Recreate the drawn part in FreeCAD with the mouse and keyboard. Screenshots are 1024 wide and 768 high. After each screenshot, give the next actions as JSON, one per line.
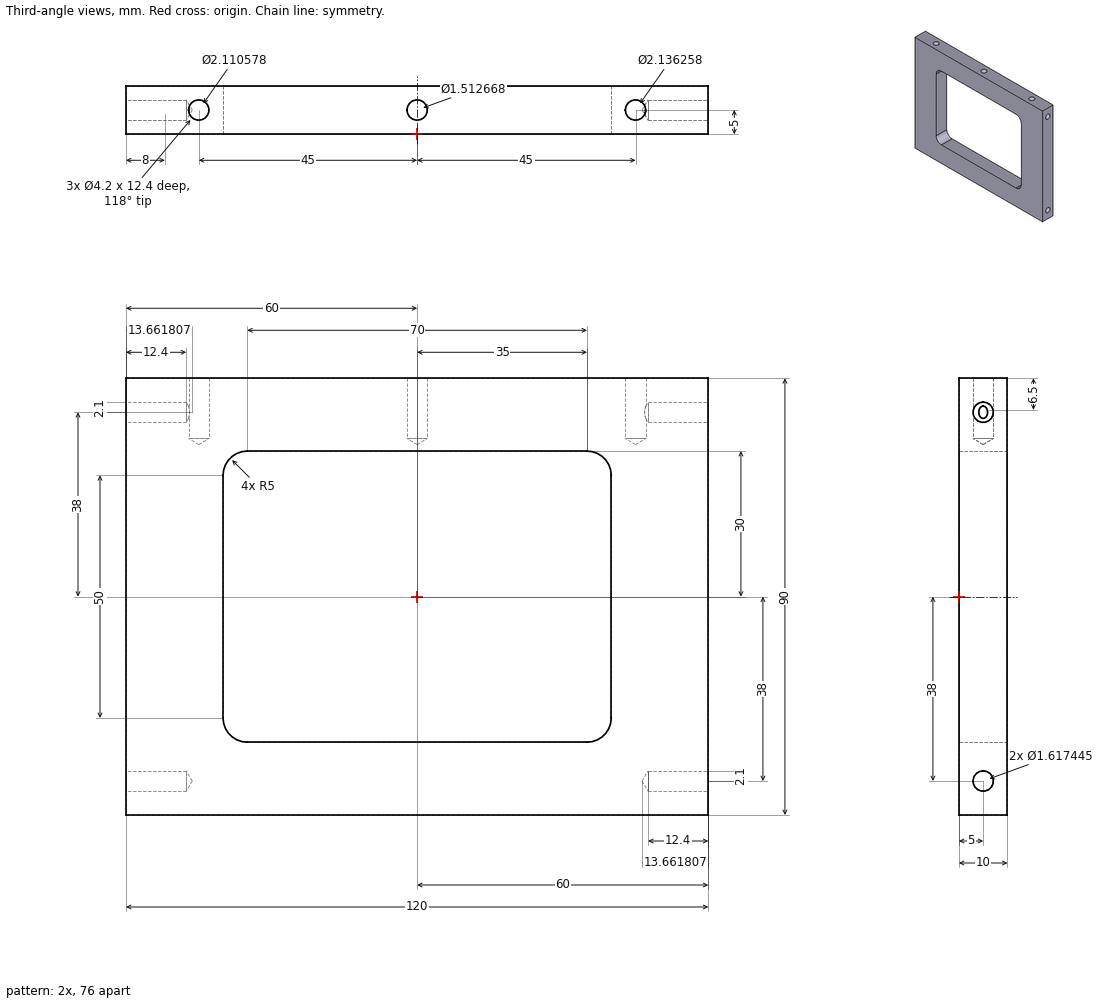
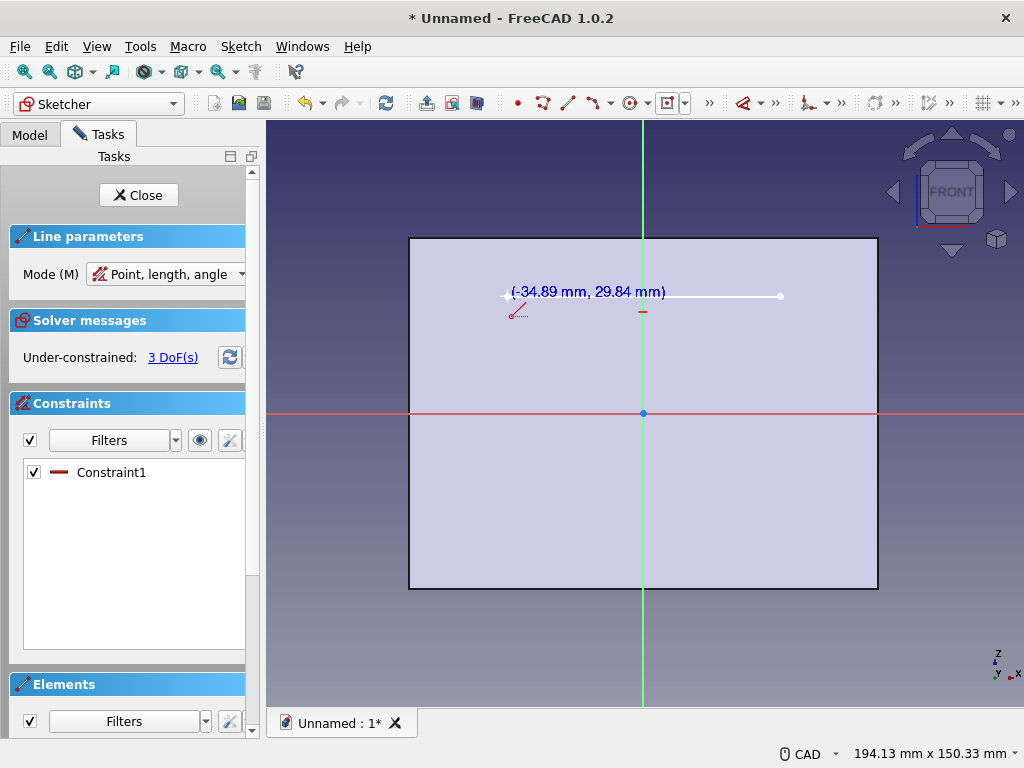
{"action": "left_click", "coordinate": [487, 316]}
{"action": "left_click", "coordinate": [487, 511]}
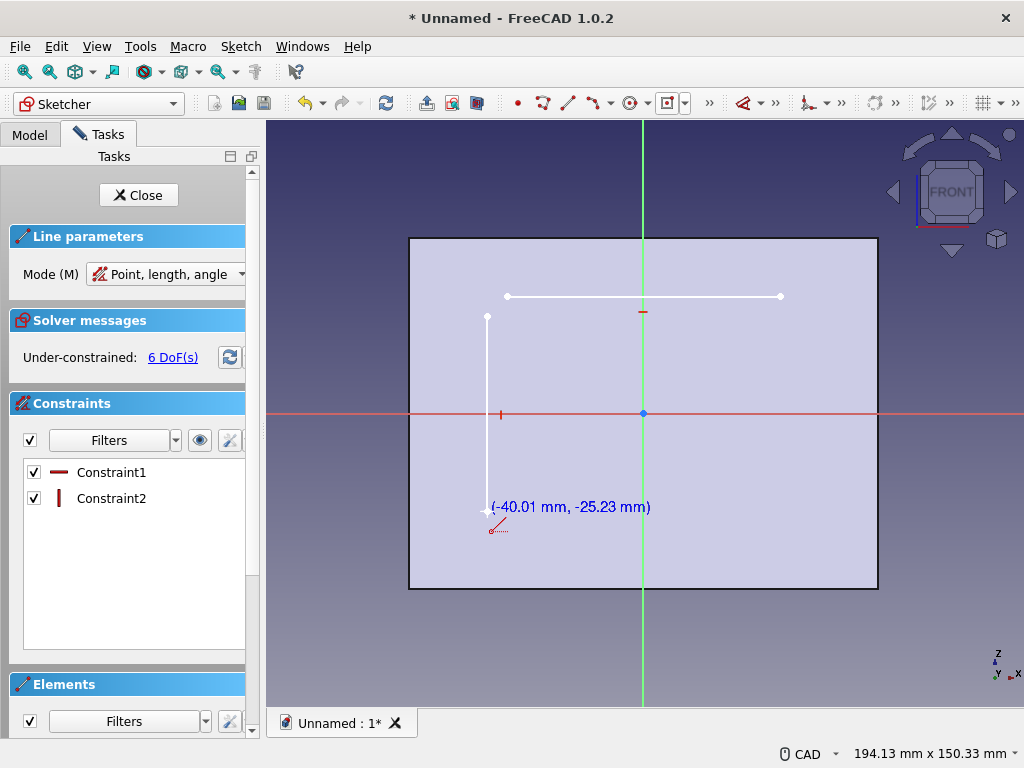
{"action": "left_click", "coordinate": [507, 531]}
{"action": "left_click", "coordinate": [780, 531]}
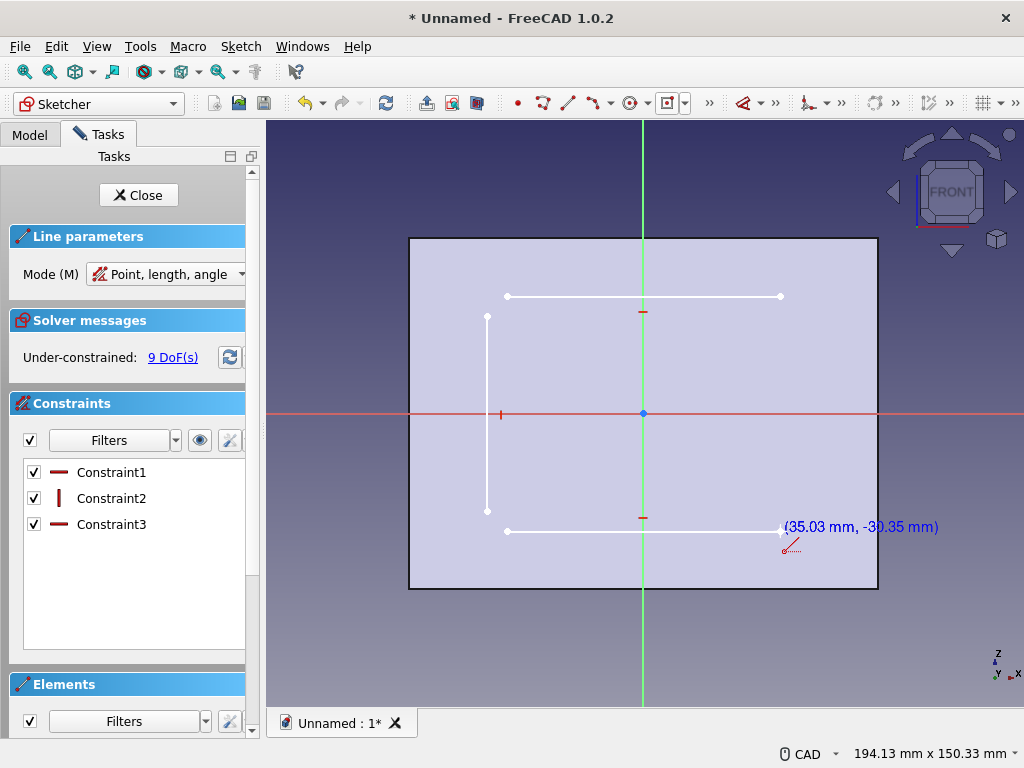
{"action": "left_click", "coordinate": [799, 511]}
{"action": "left_click", "coordinate": [799, 316]}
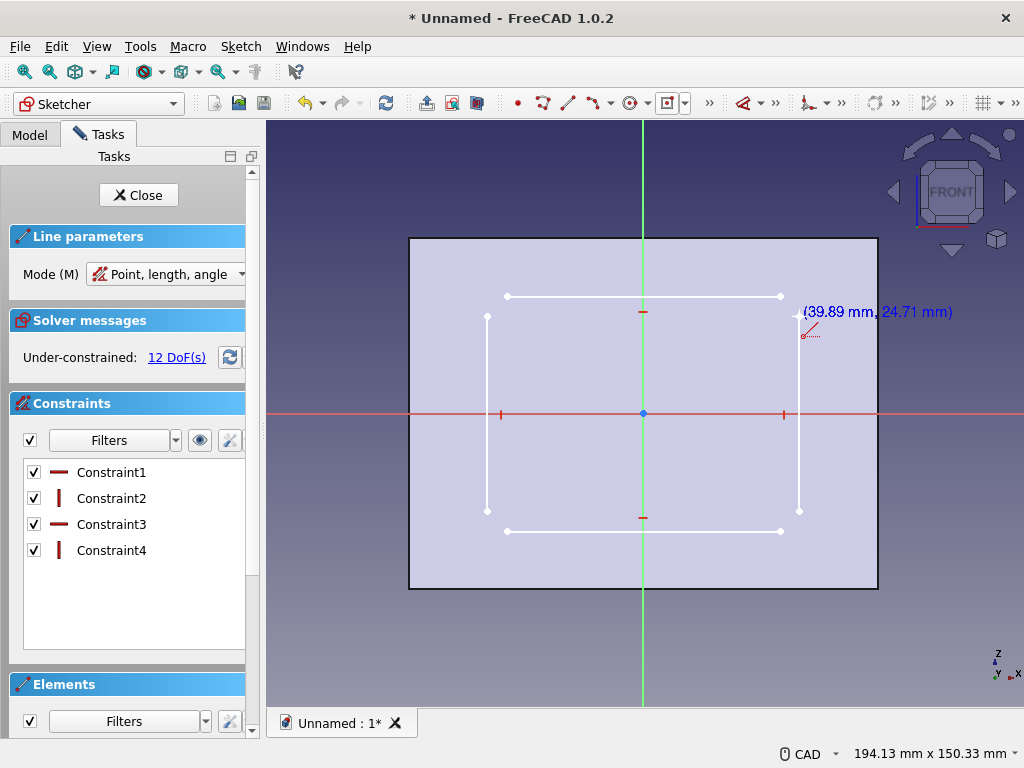
{"action": "left_click", "coordinate": [592, 104]}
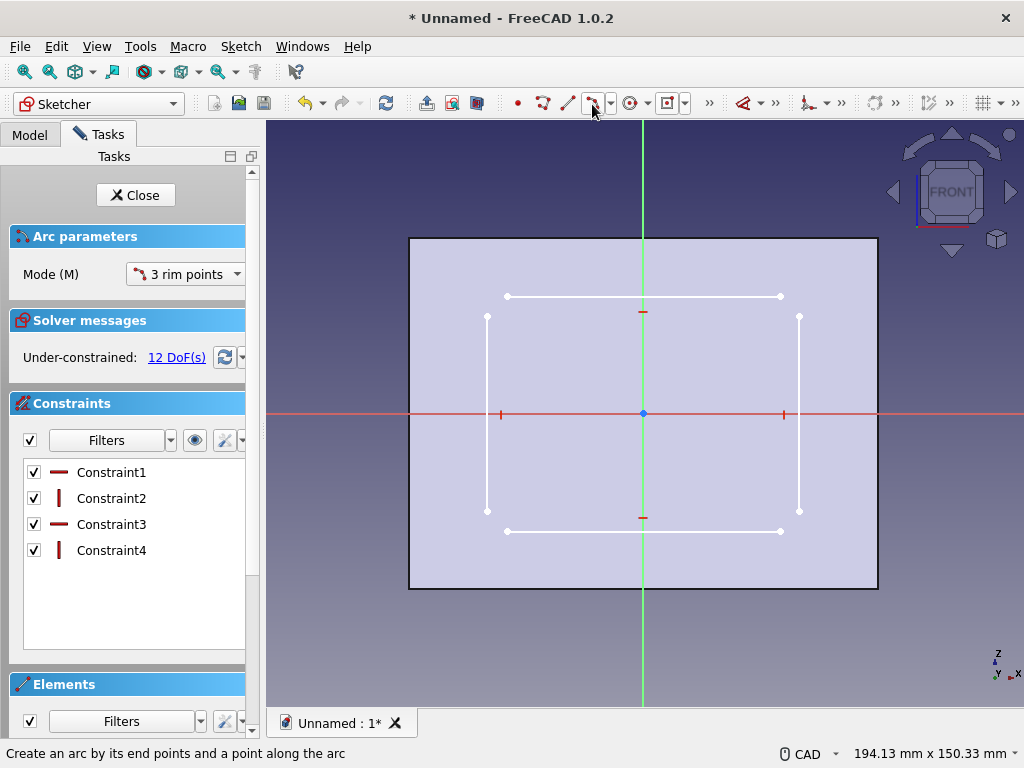
{"action": "left_click", "coordinate": [507, 297]}
{"action": "left_click", "coordinate": [487, 317]}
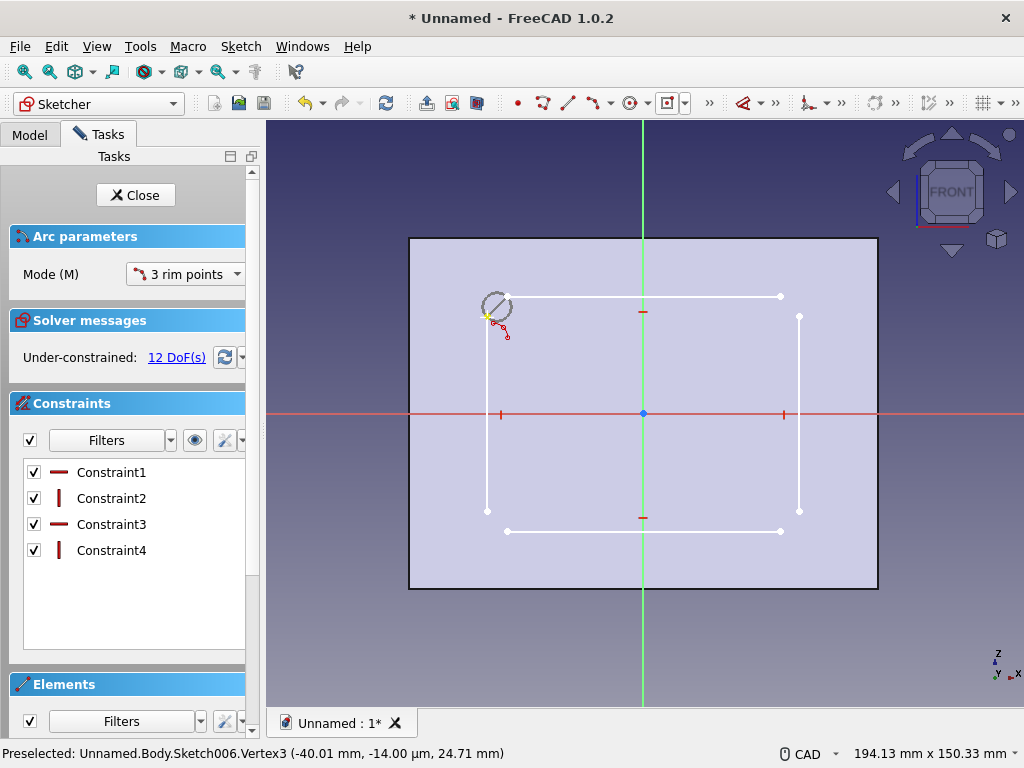
{"action": "scroll", "coordinate": [493, 302], "scroll_direction": "up", "scroll_amount": 6}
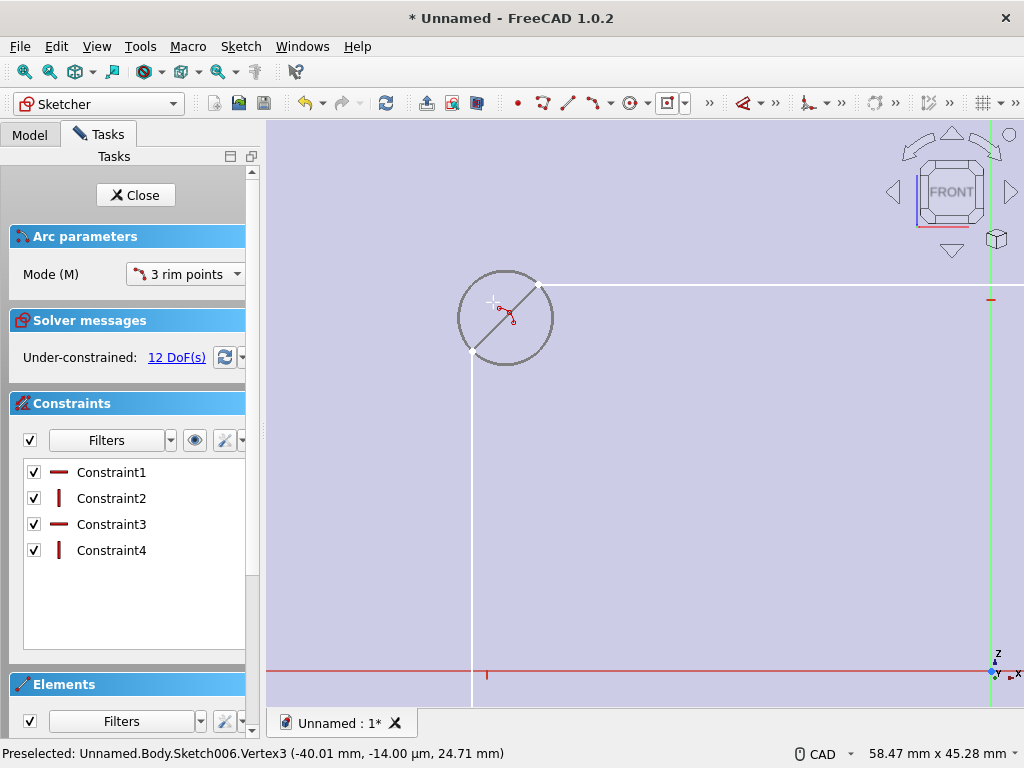
{"action": "left_click", "coordinate": [492, 302]}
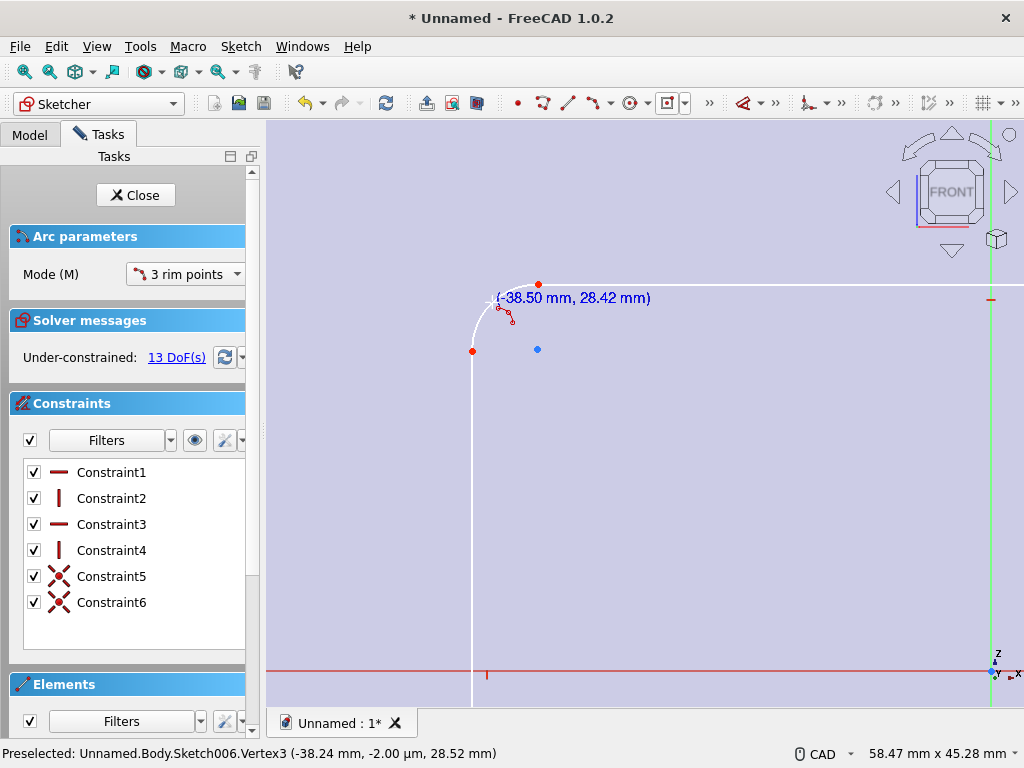
{"action": "scroll", "coordinate": [335, 263], "scroll_direction": "down", "scroll_amount": 5}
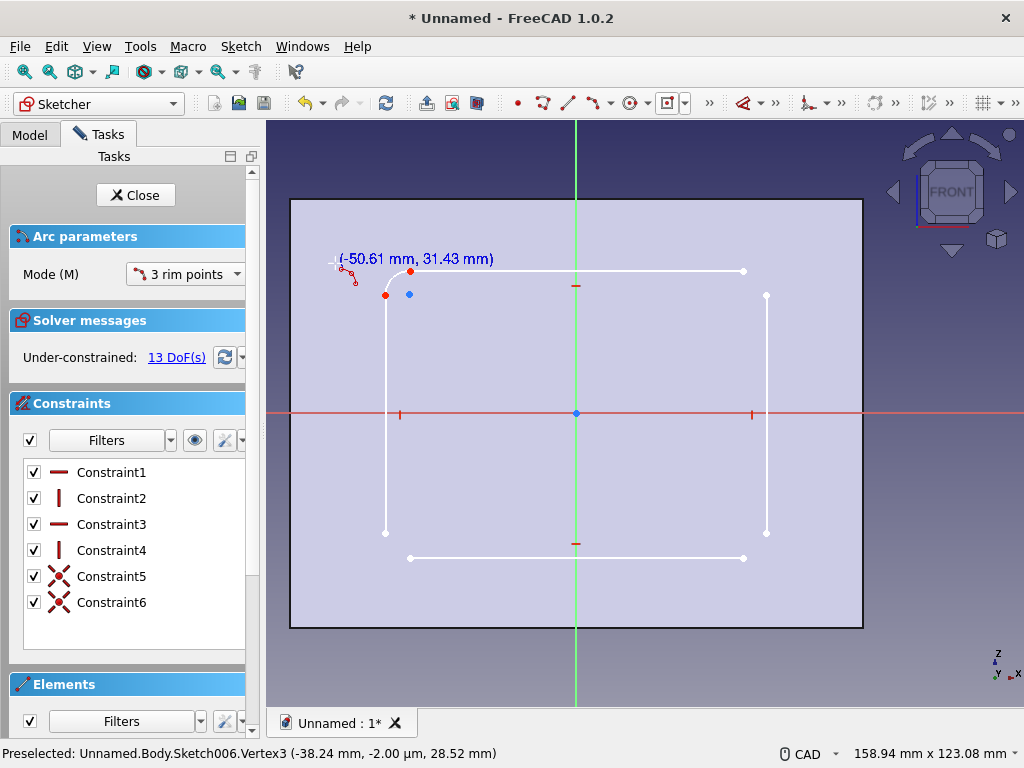
{"action": "left_click", "coordinate": [386, 534]}
{"action": "left_click", "coordinate": [410, 558]}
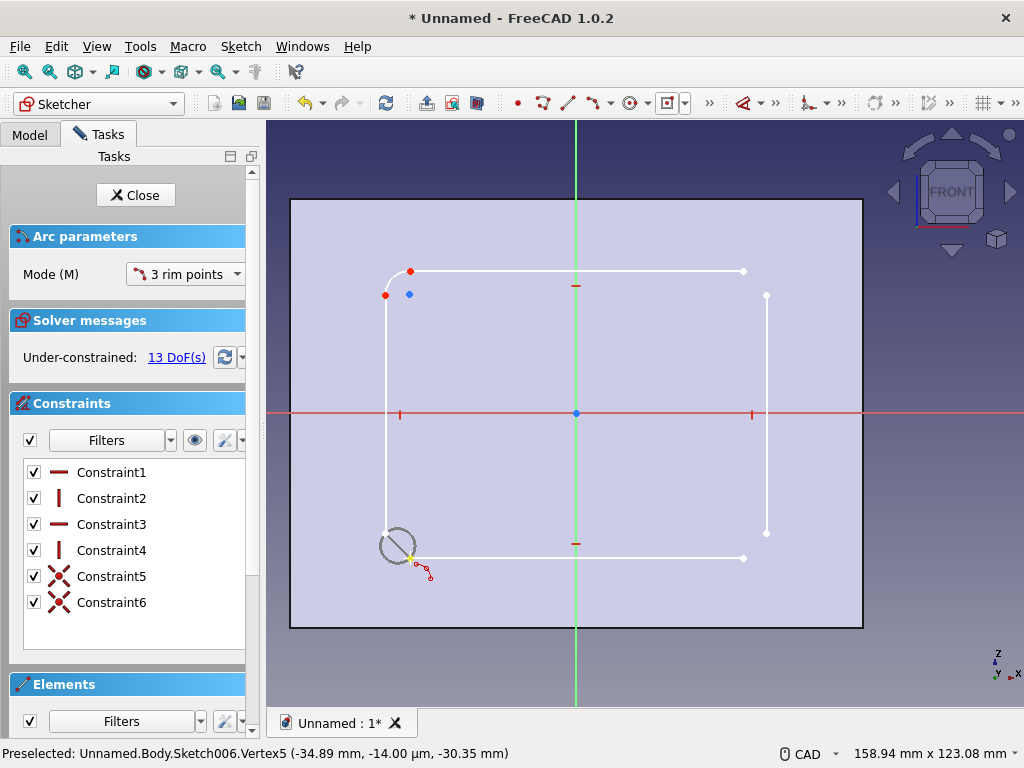
{"action": "scroll", "coordinate": [393, 550], "scroll_direction": "up", "scroll_amount": 5}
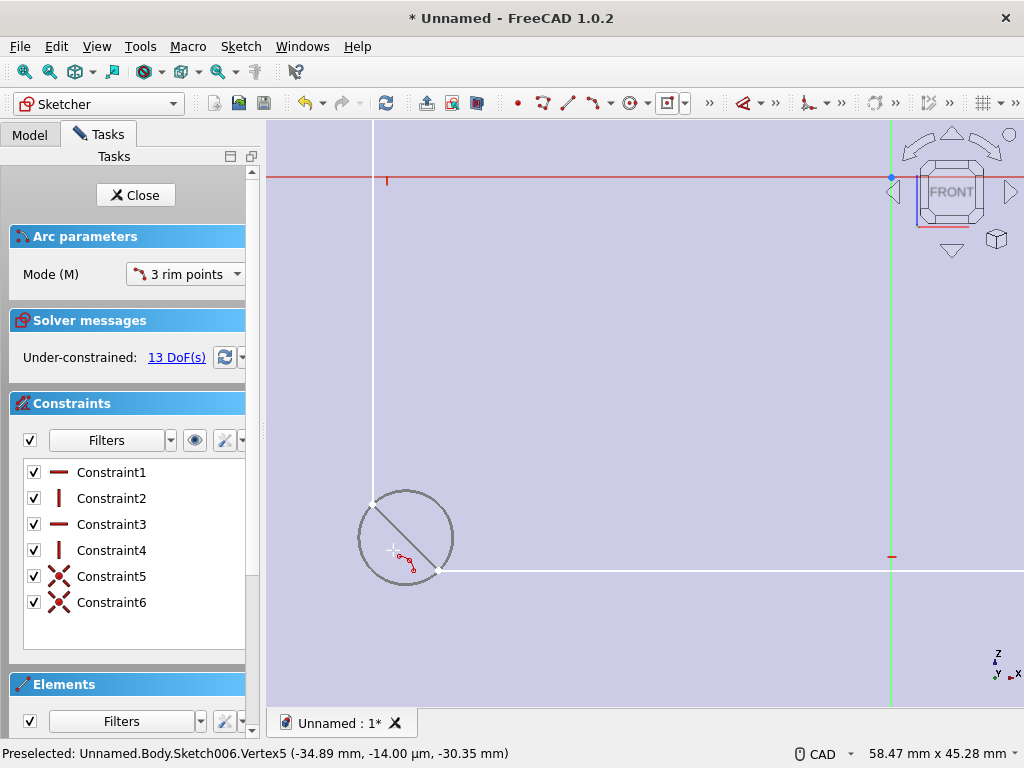
{"action": "left_click", "coordinate": [392, 547]}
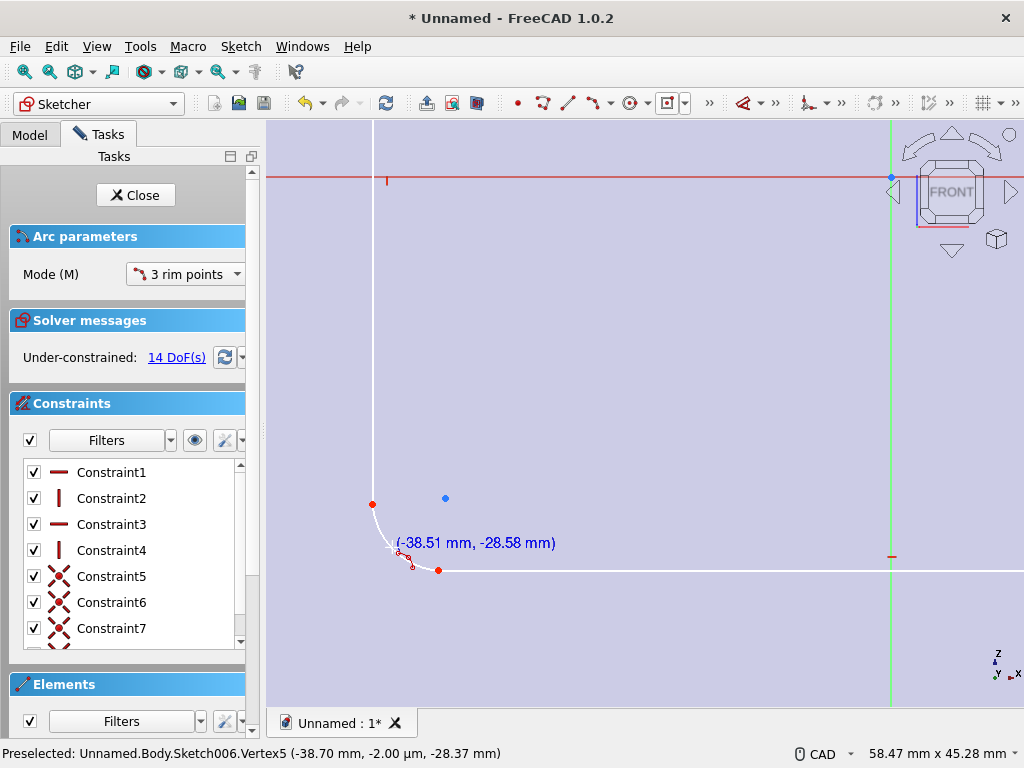
{"action": "scroll", "coordinate": [393, 551], "scroll_direction": "down", "scroll_amount": 5}